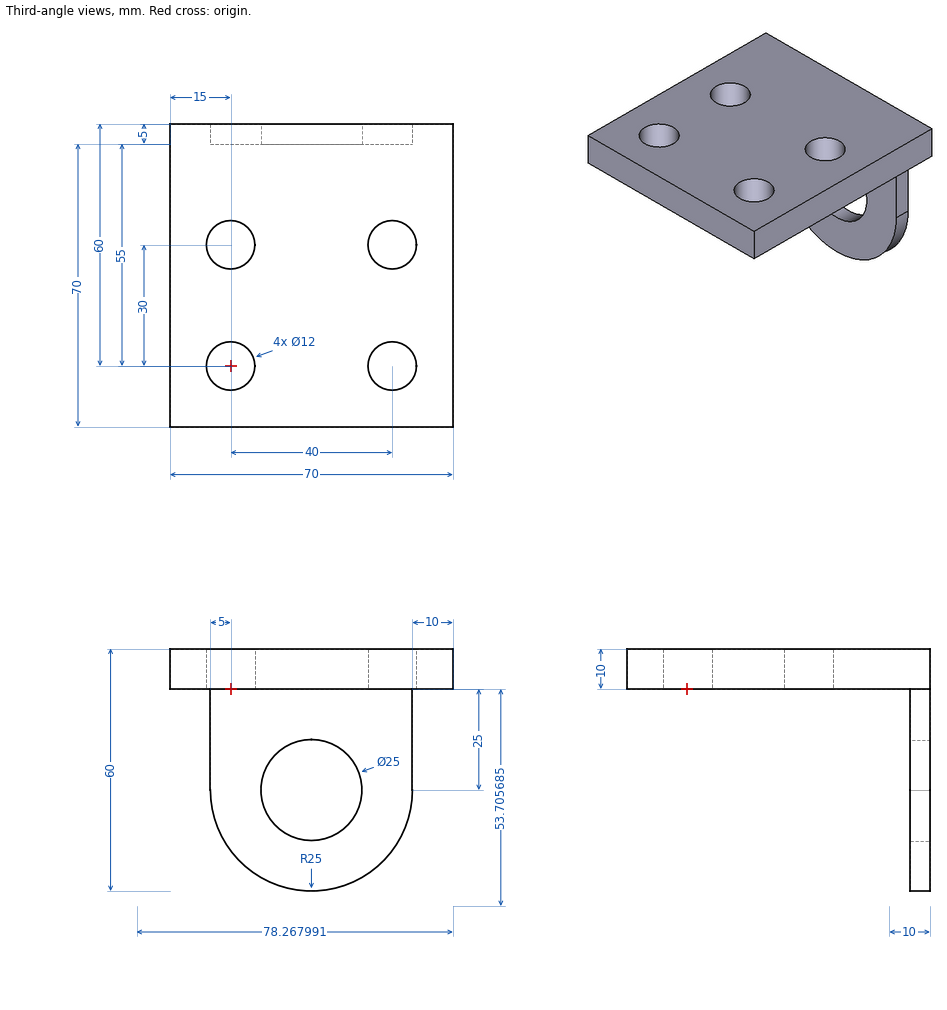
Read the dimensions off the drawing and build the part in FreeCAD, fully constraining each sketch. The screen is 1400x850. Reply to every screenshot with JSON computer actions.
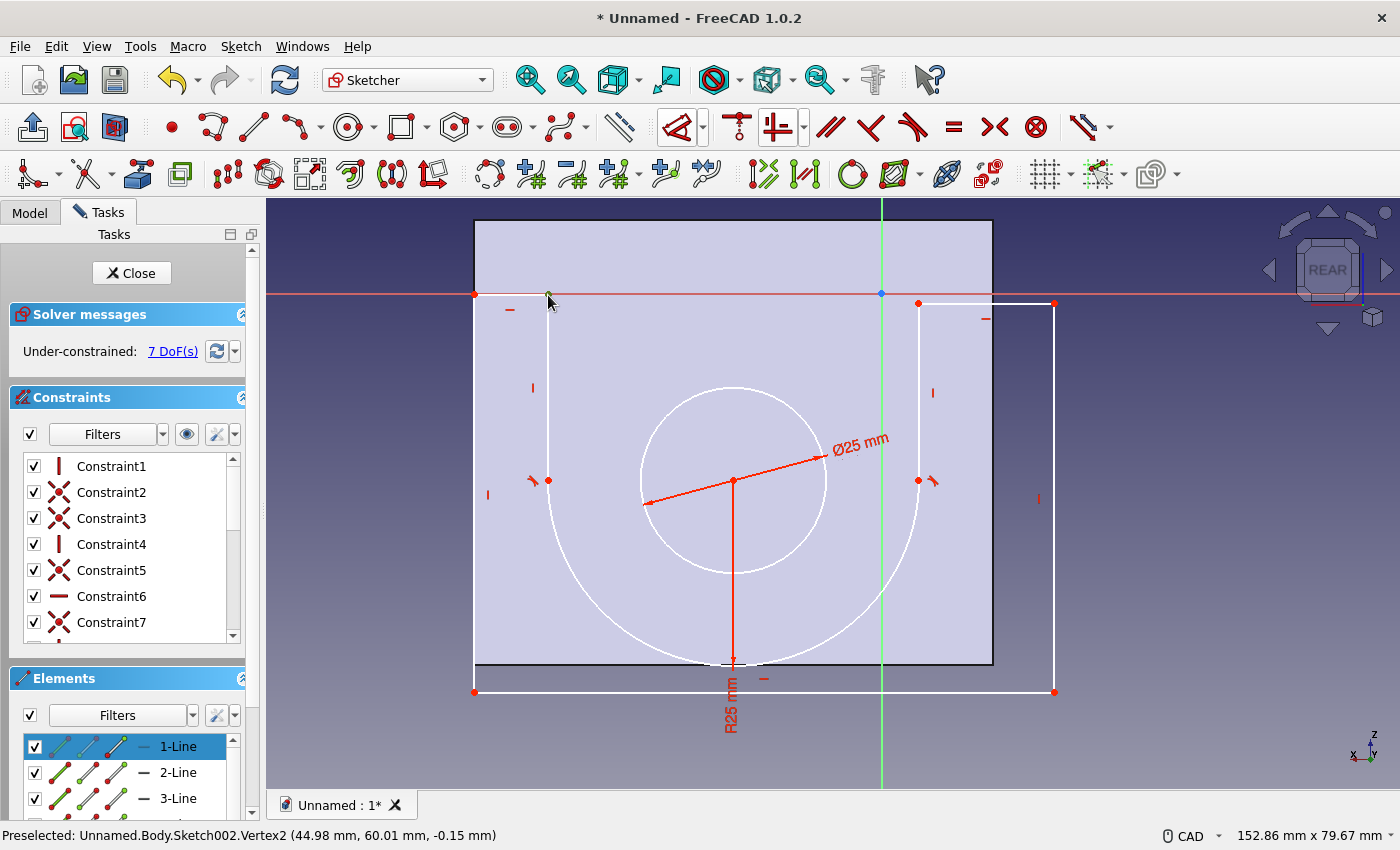
{"action": "left_click", "coordinate": [361, 294]}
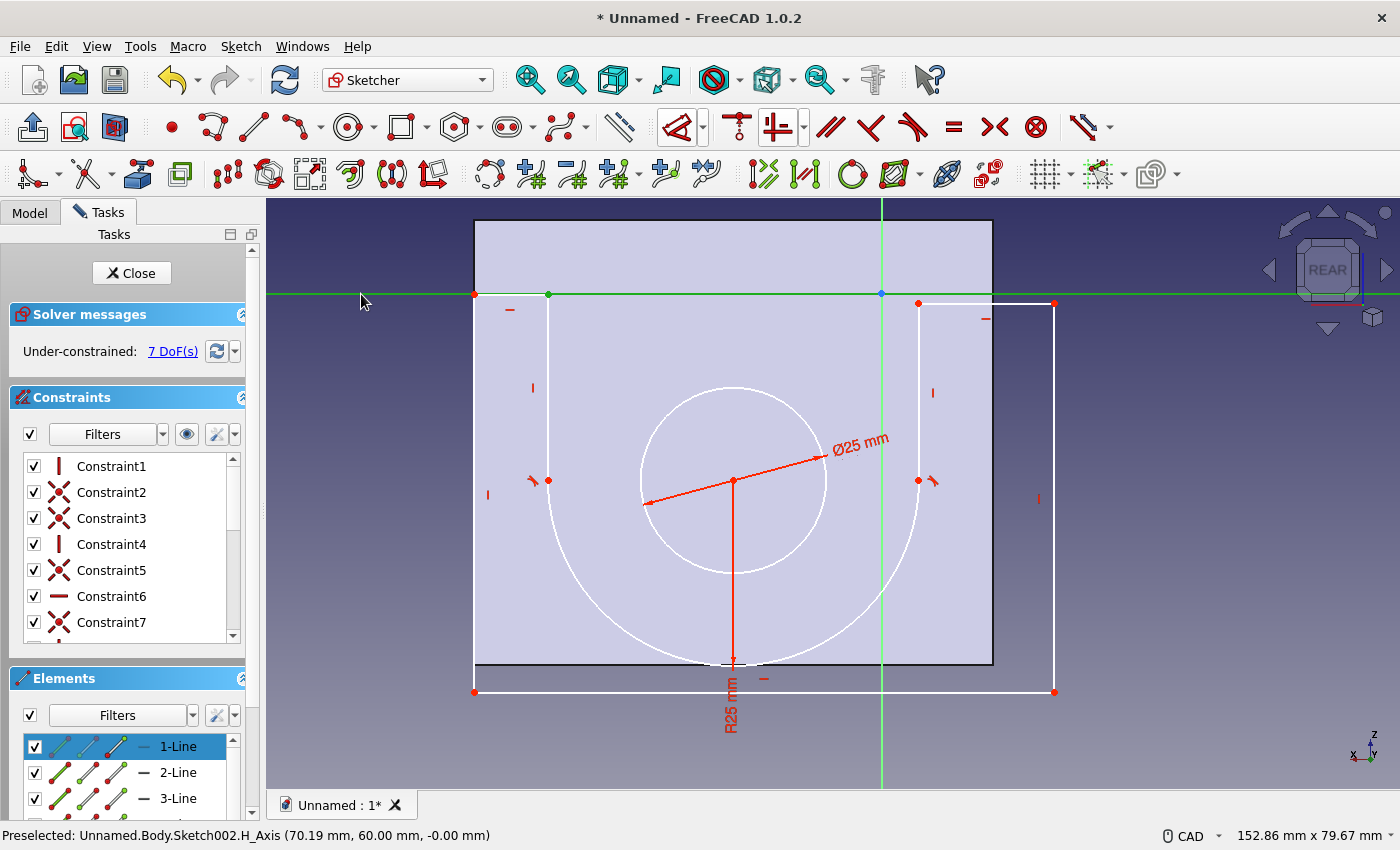
{"action": "key", "text": "c"}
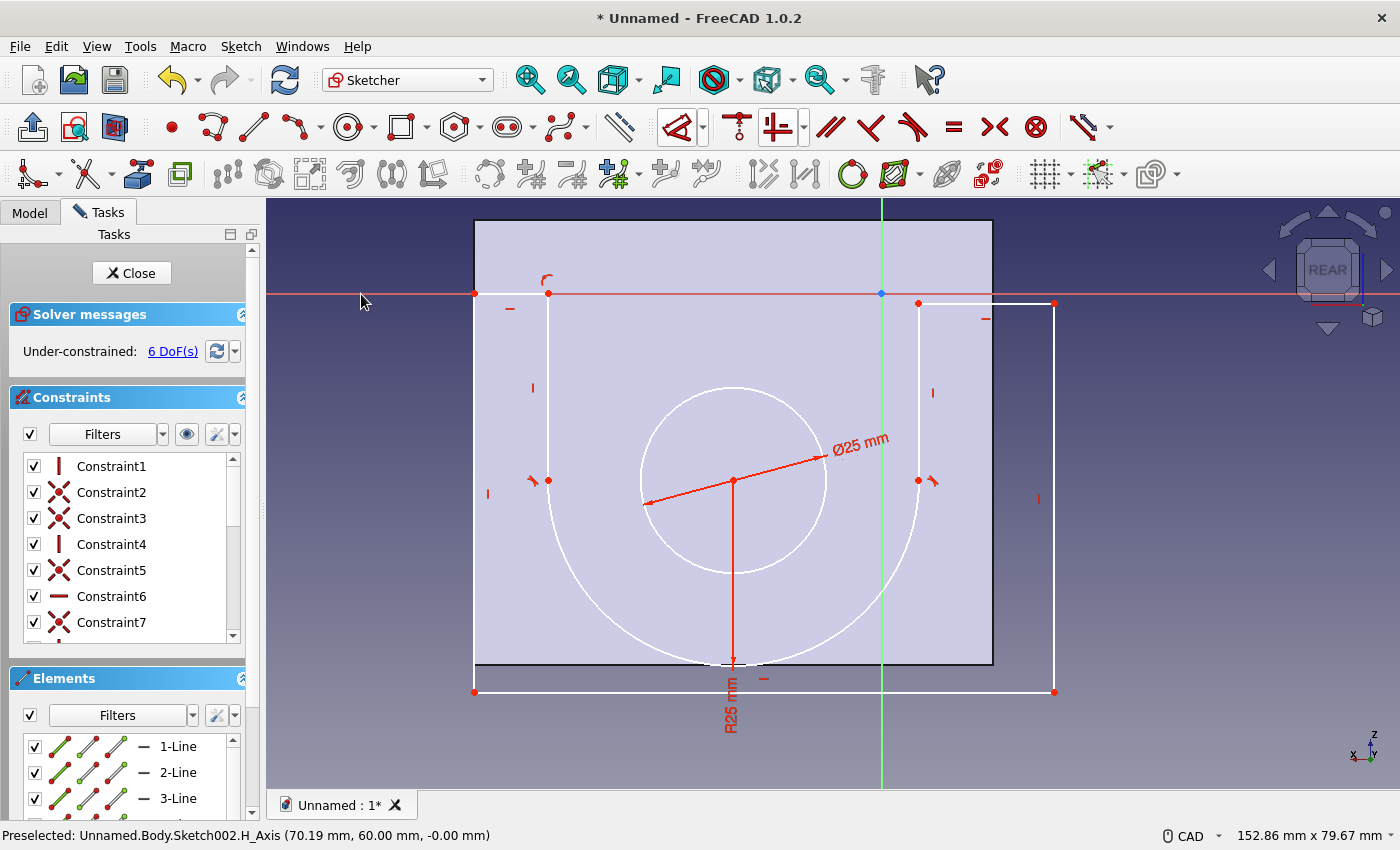
{"action": "left_click", "coordinate": [1054, 304]}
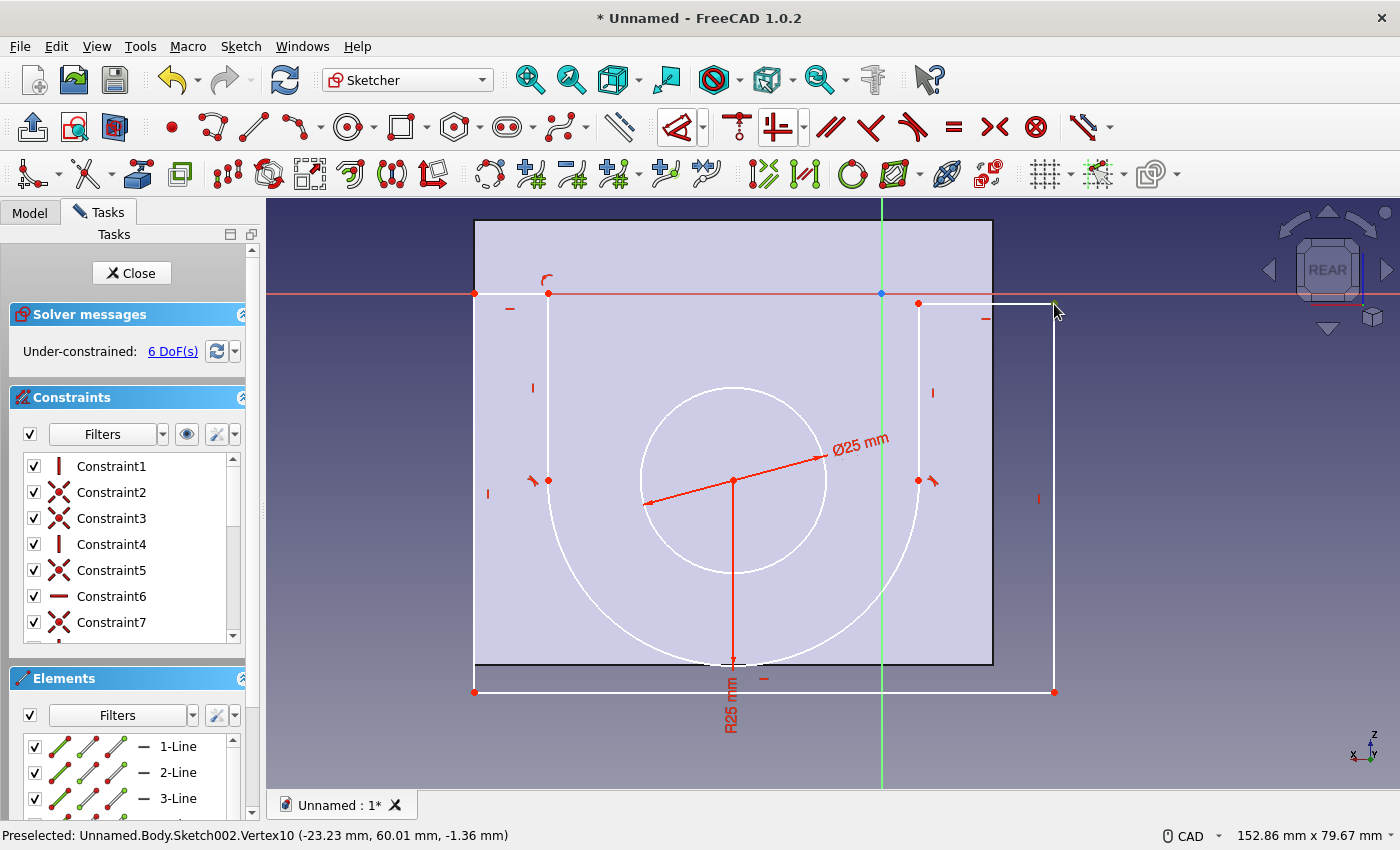
{"action": "left_click", "coordinate": [361, 294]}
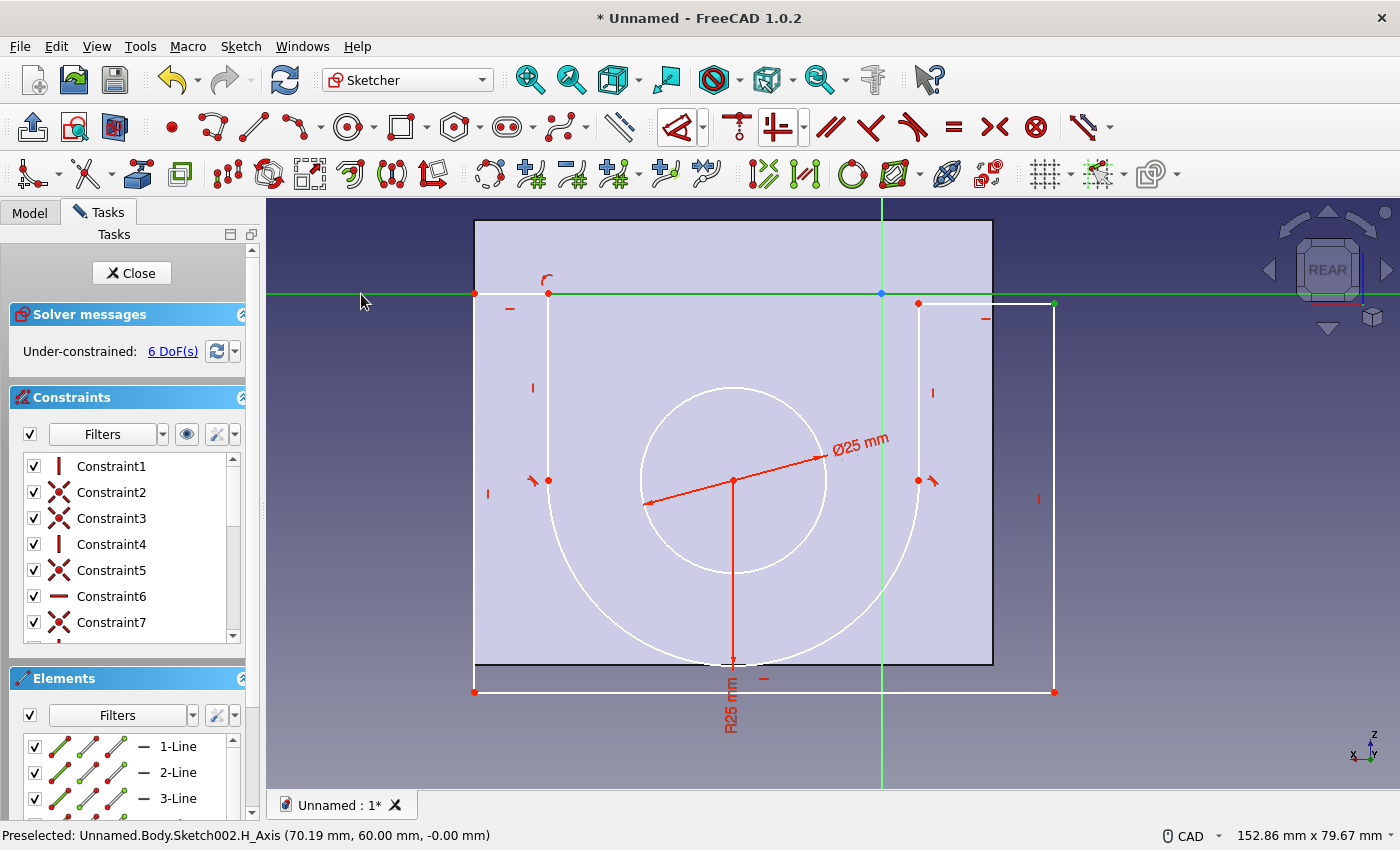
{"action": "left_click", "coordinate": [737, 128]}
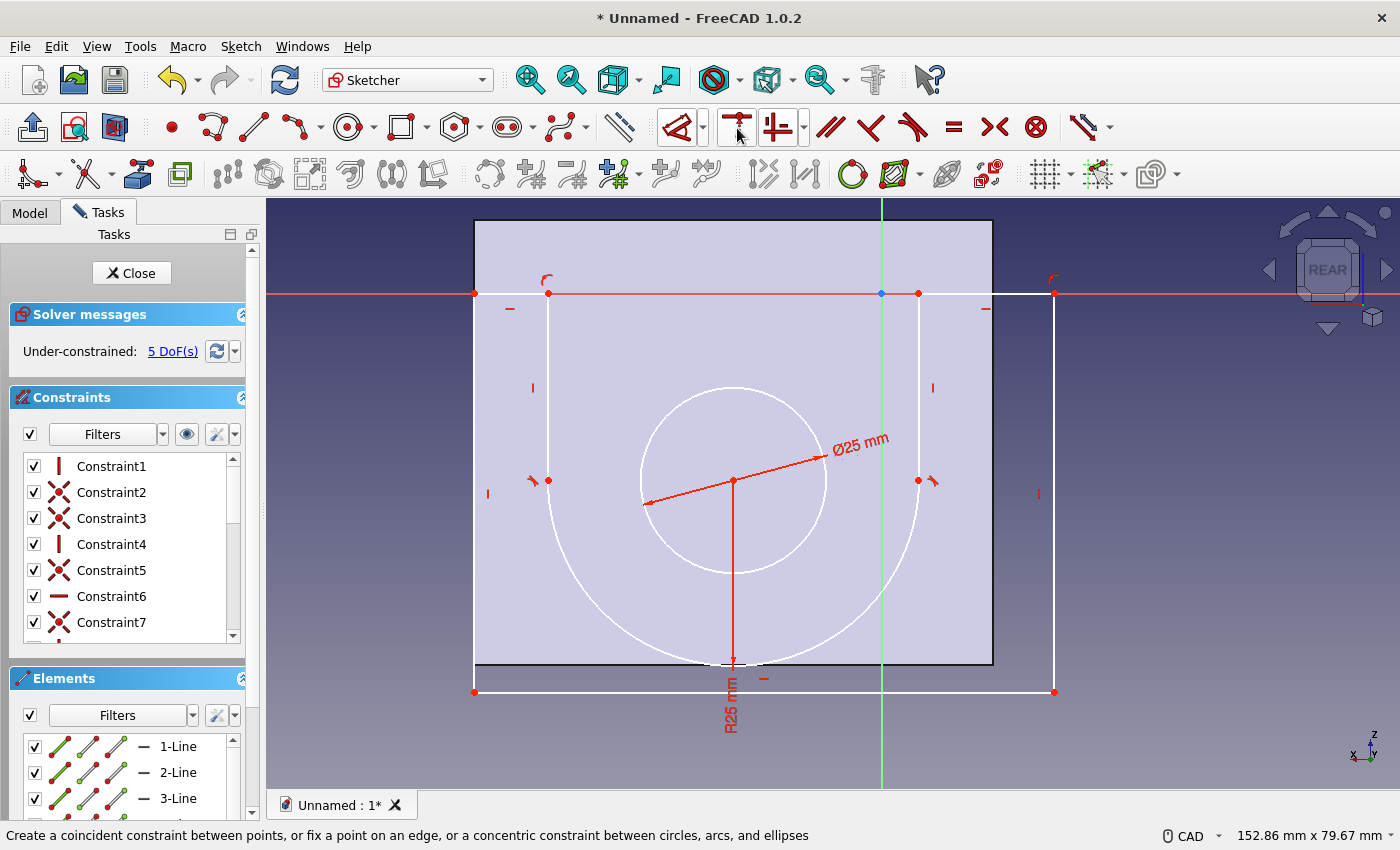
{"action": "left_click", "coordinate": [548, 425]}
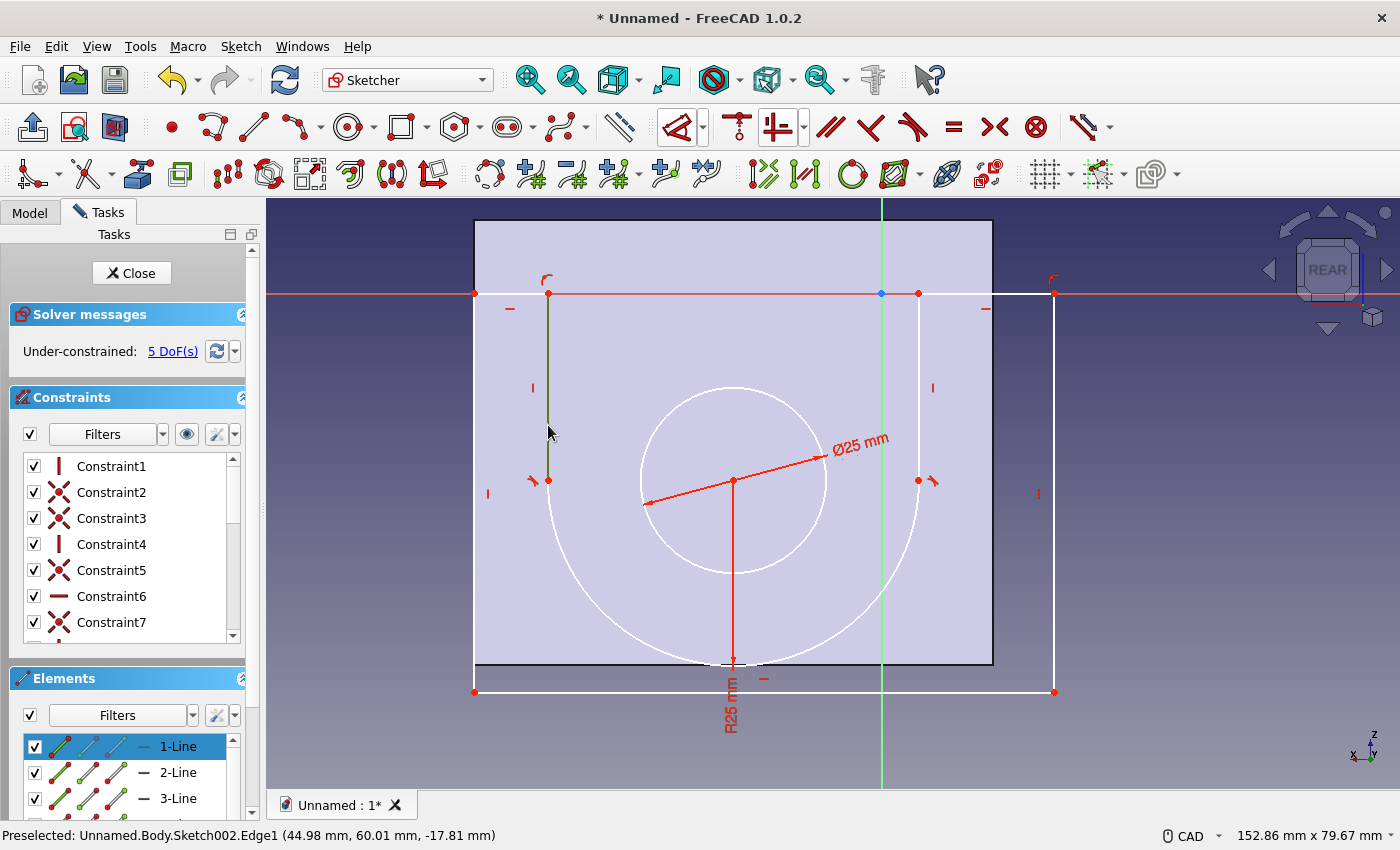
{"action": "key", "text": "i"}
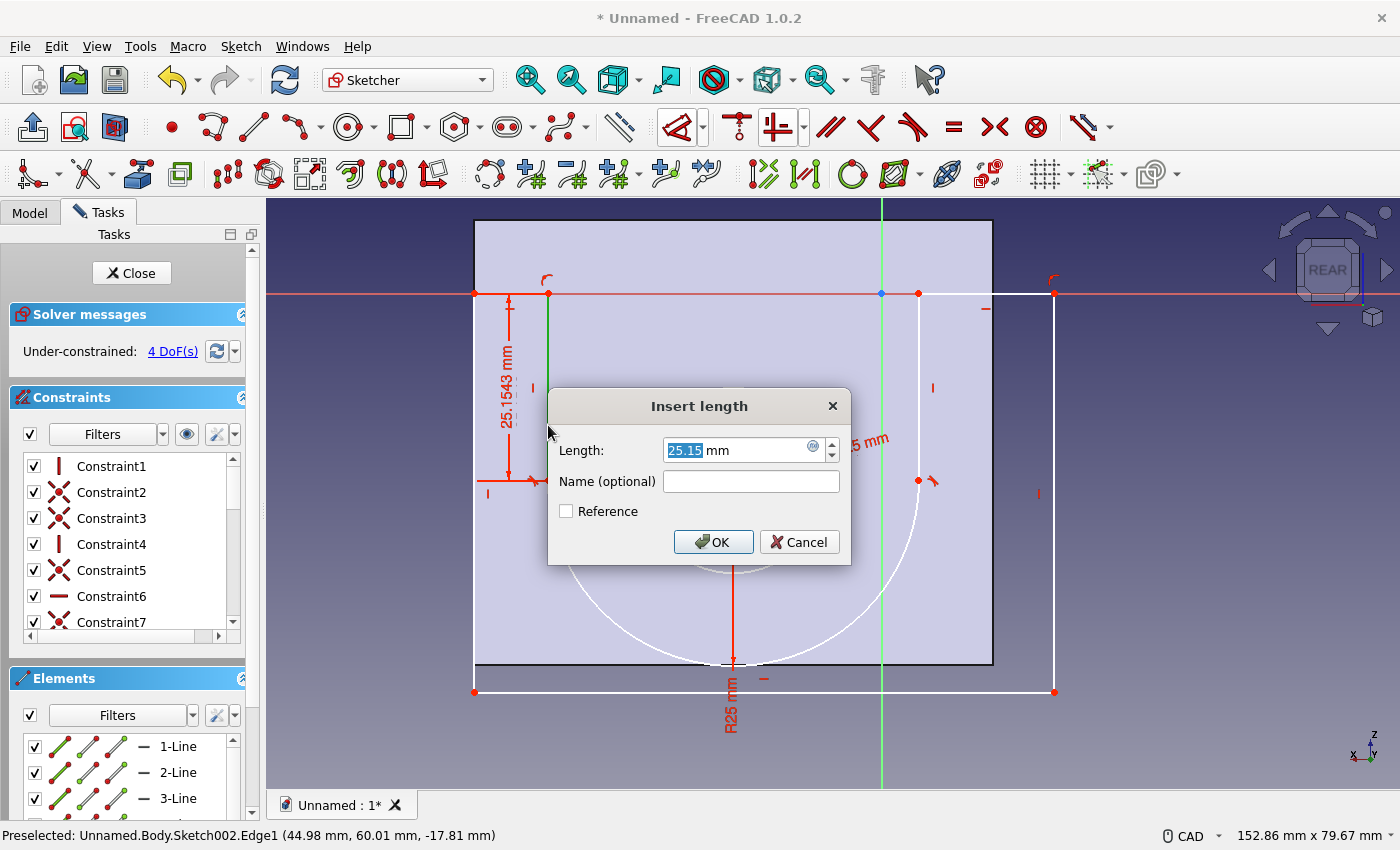
{"action": "type", "text": "25"}
{"action": "key", "text": "Return"}